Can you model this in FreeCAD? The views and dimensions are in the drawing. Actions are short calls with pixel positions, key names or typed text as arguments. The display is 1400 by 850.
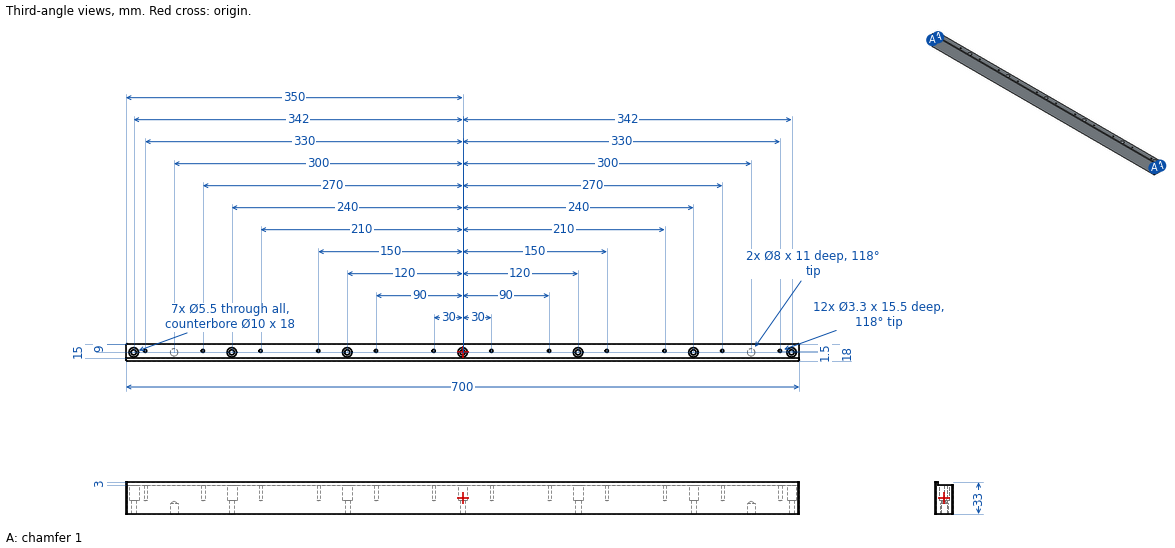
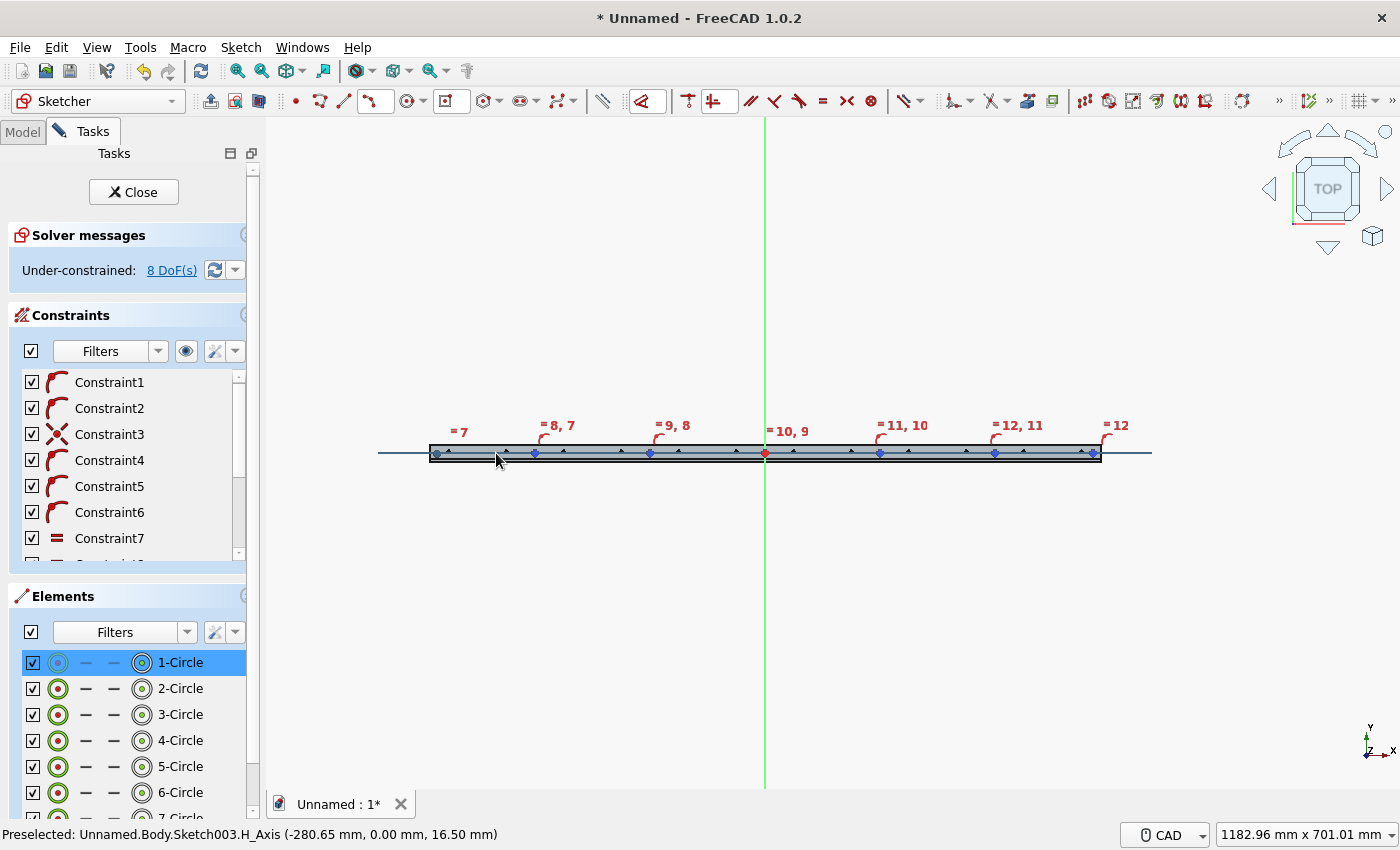
key(c)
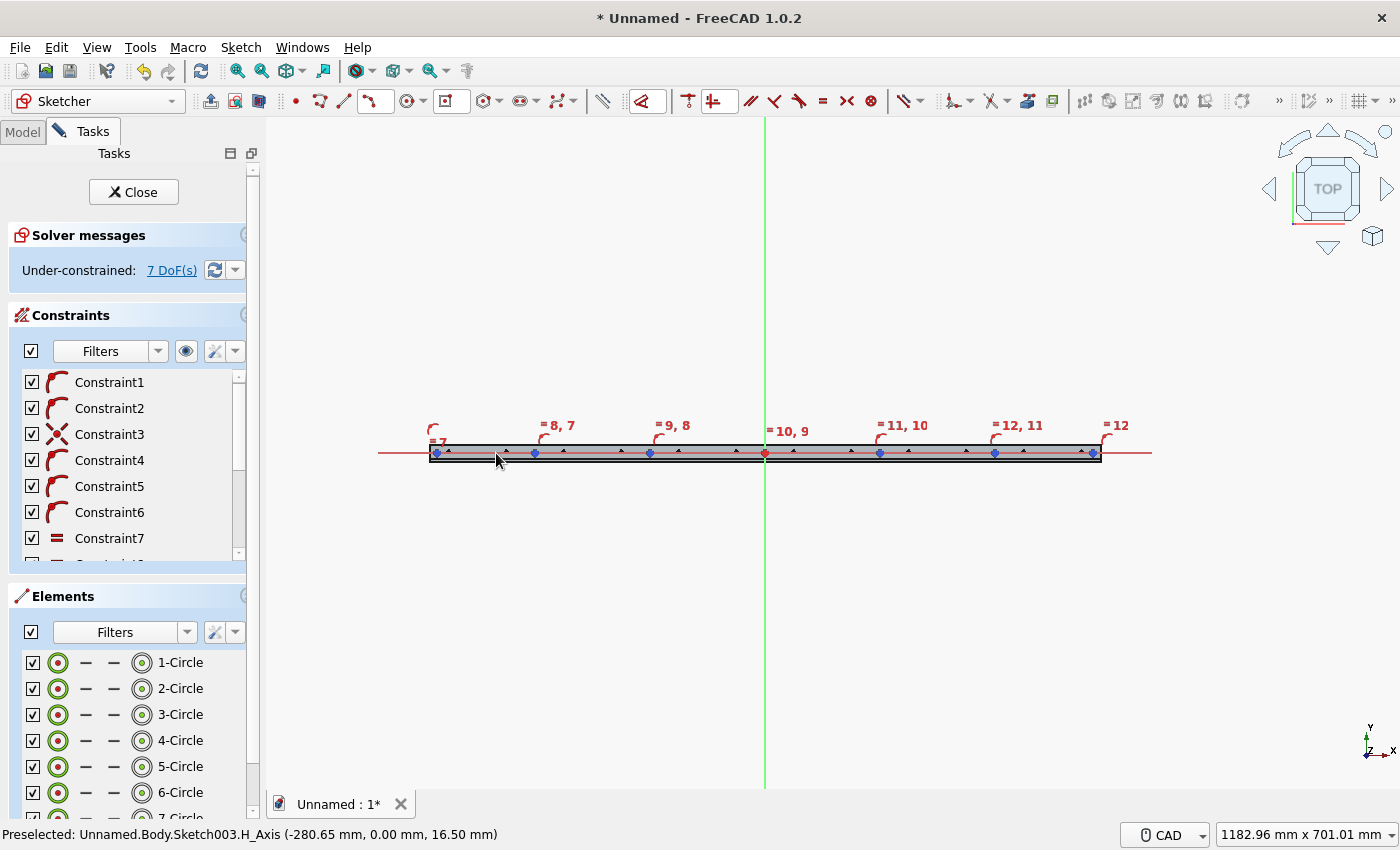
scroll(435, 456, up, 11)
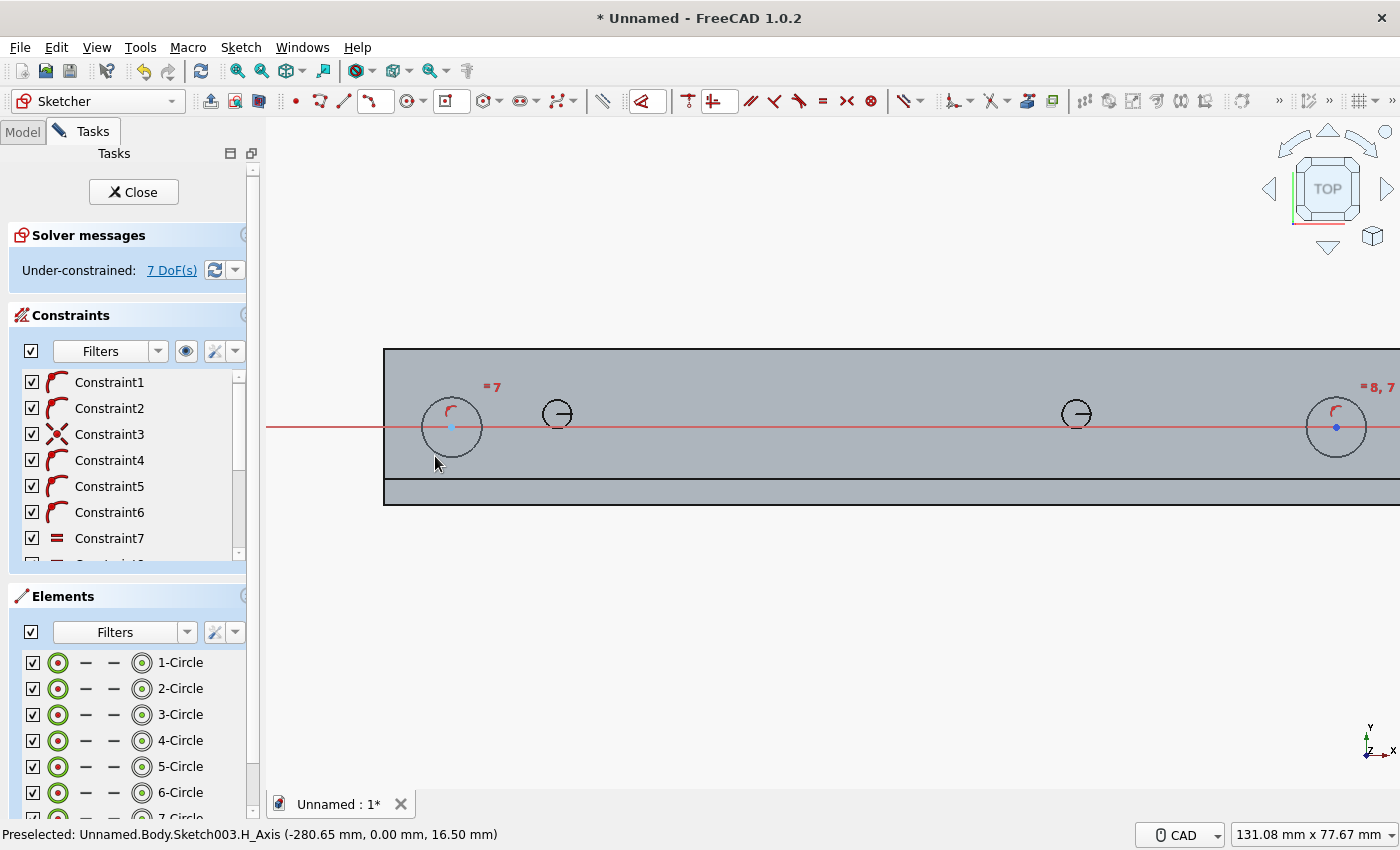
click(431, 448)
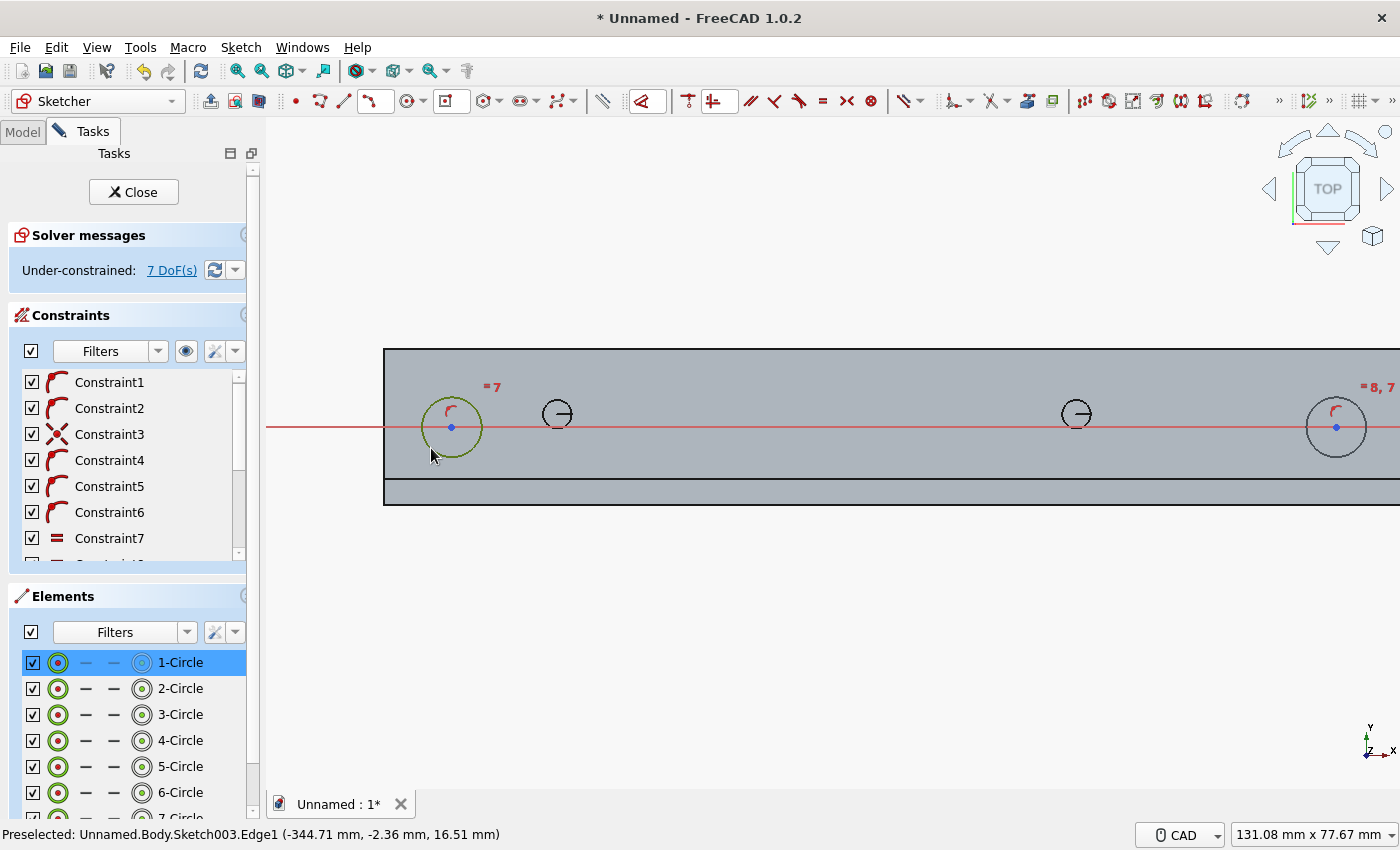
key(k)
key(o)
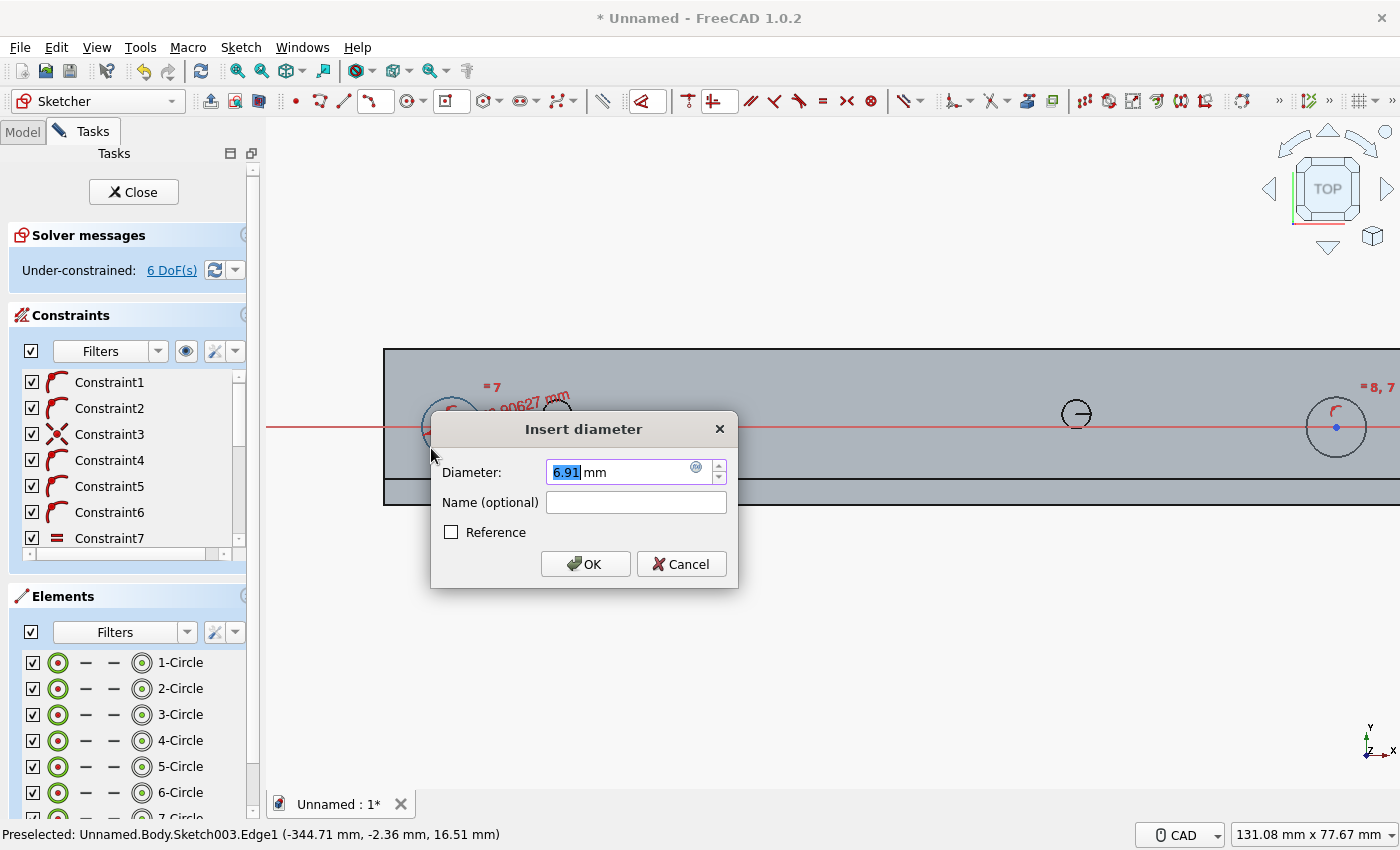
text(5.5)
key(Return)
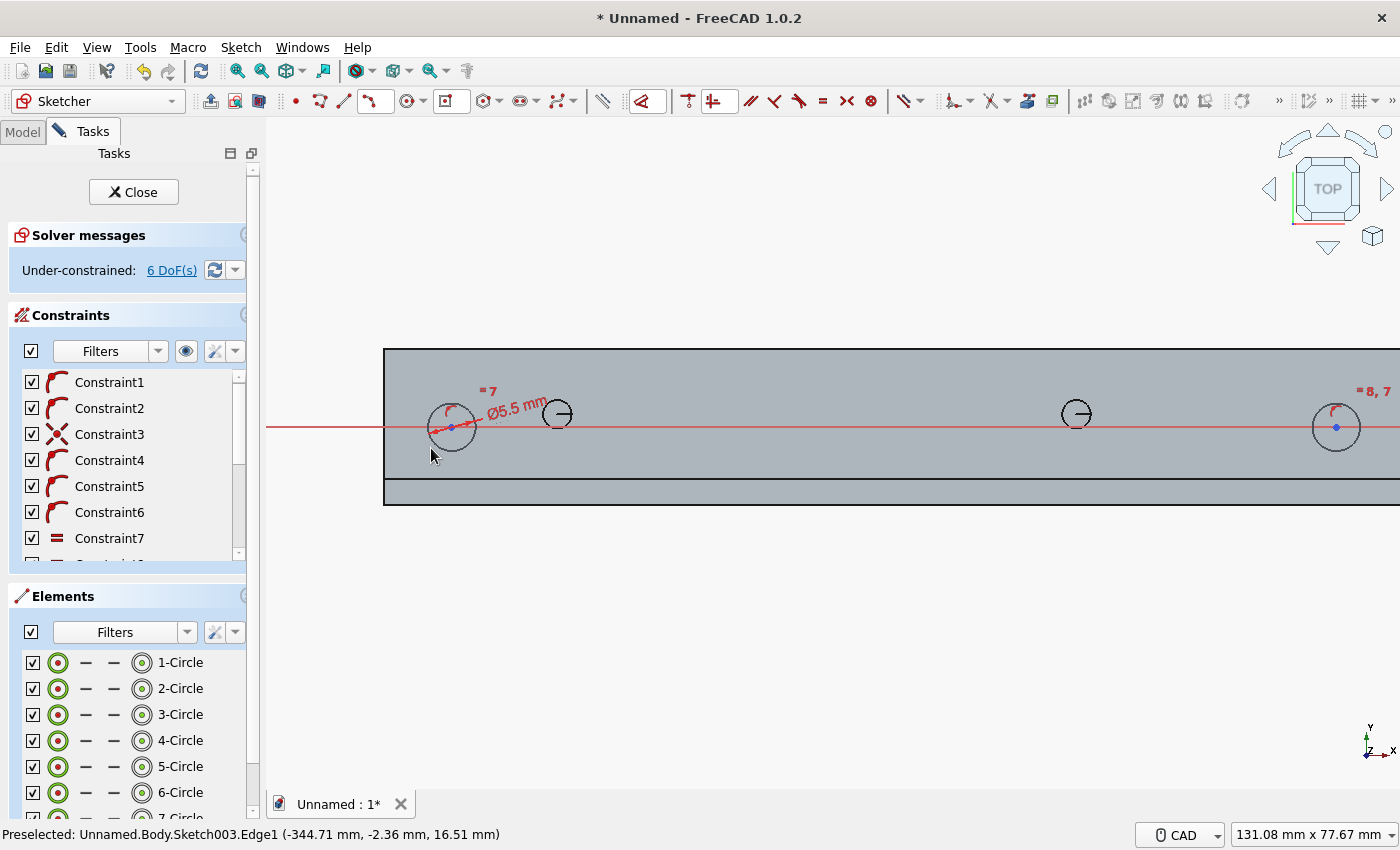
scroll(435, 456, down, 11)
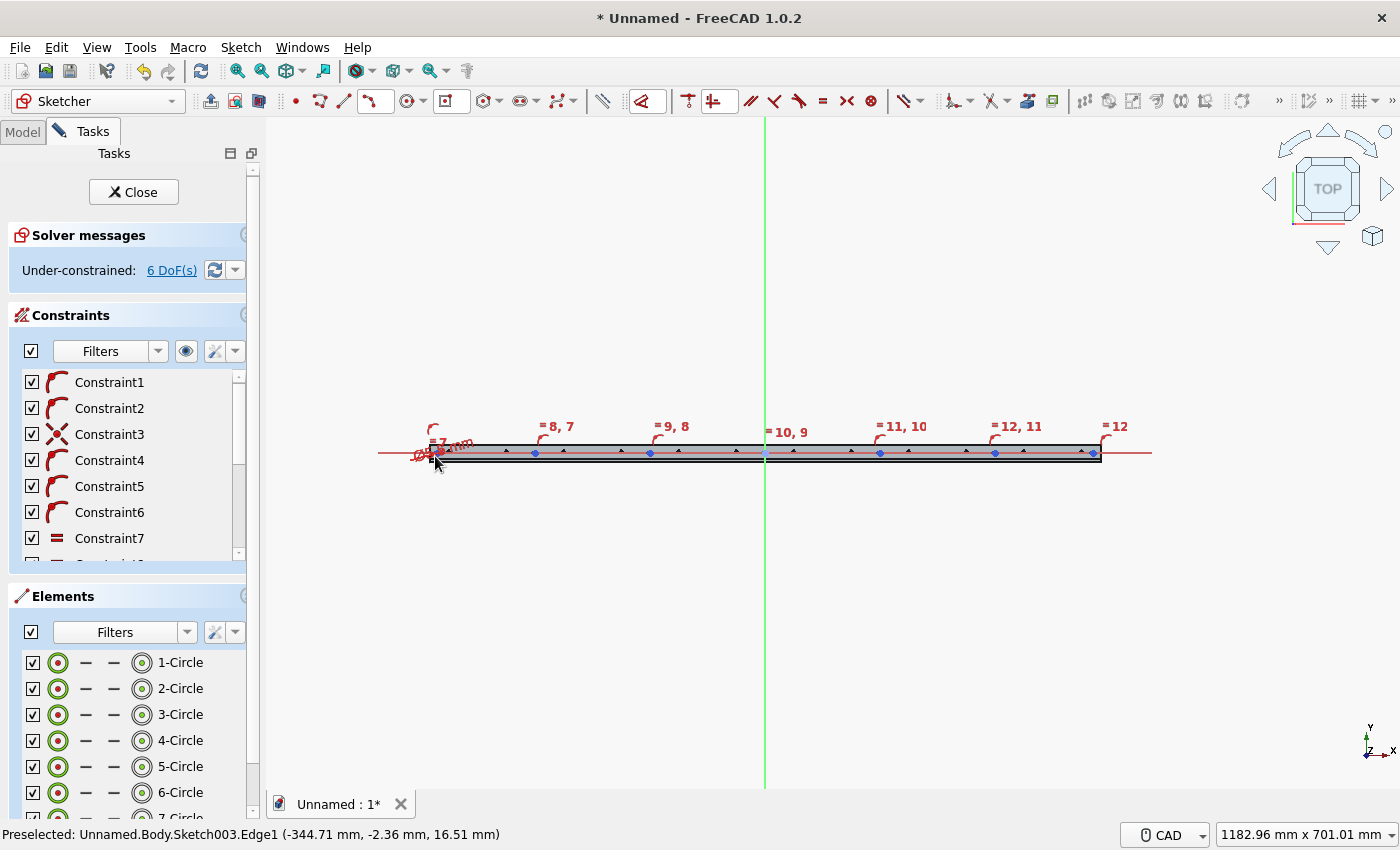
click(437, 453)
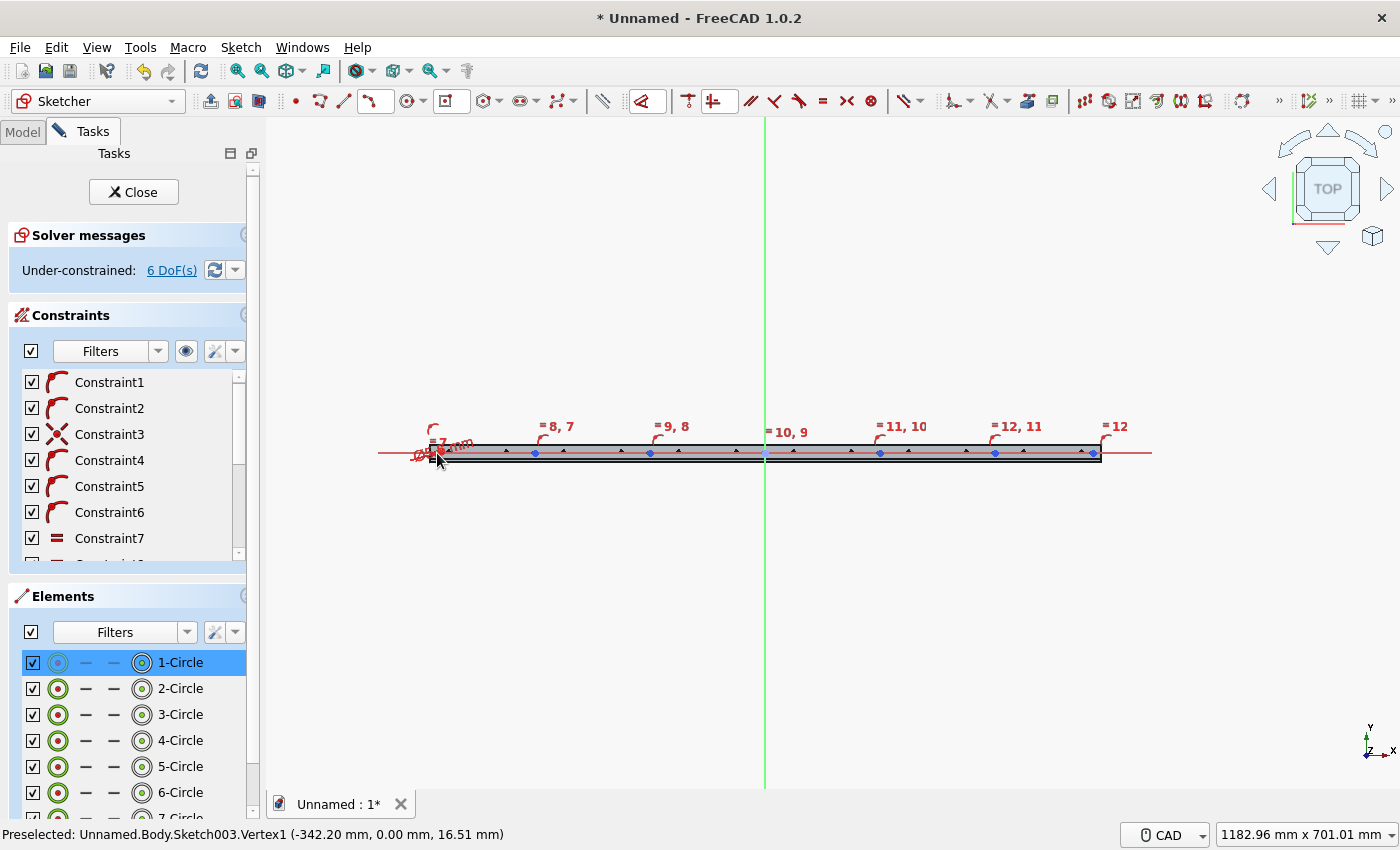
key(l)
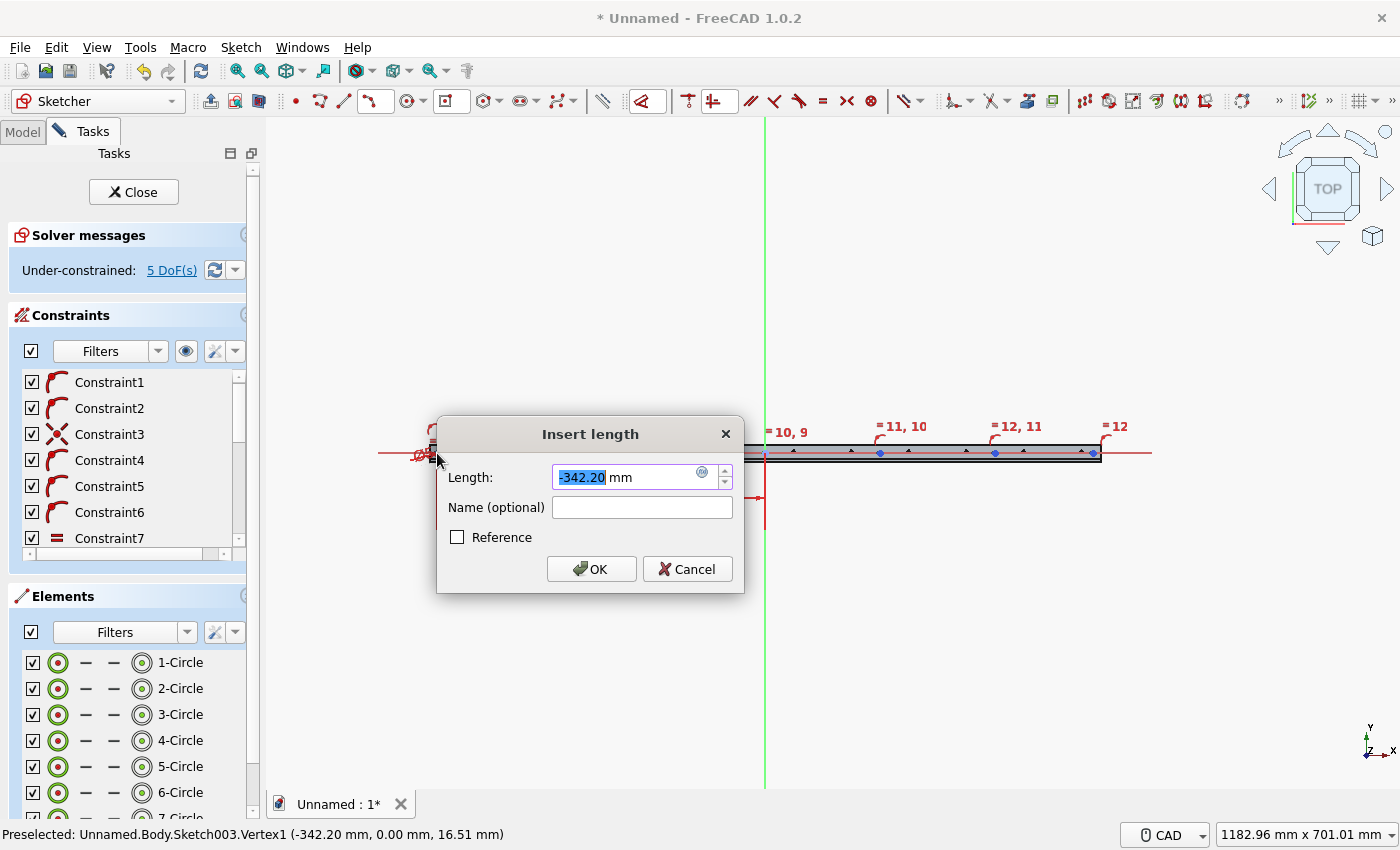
text(-342)
key(Return)